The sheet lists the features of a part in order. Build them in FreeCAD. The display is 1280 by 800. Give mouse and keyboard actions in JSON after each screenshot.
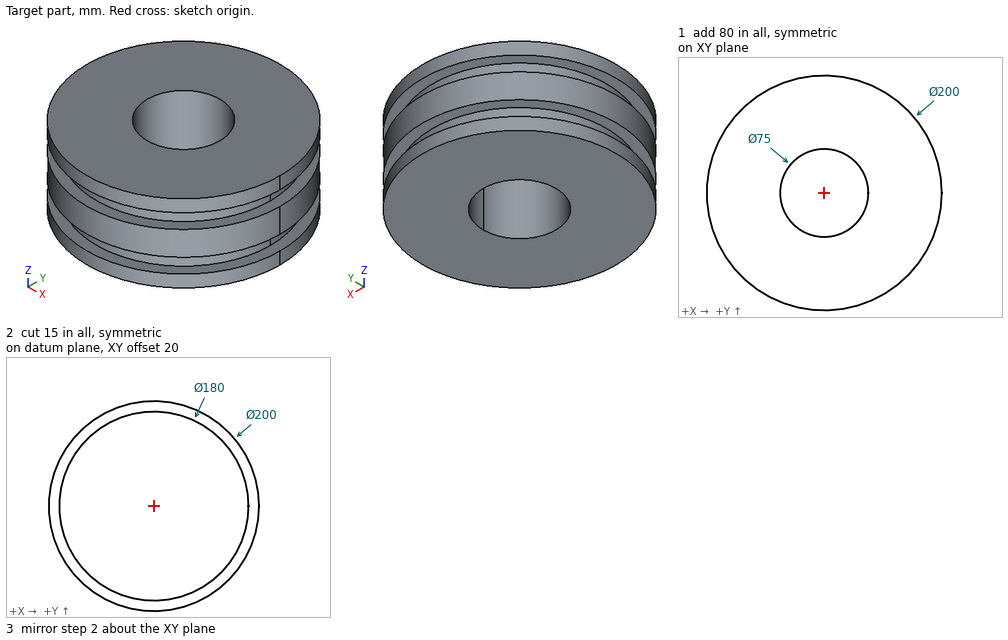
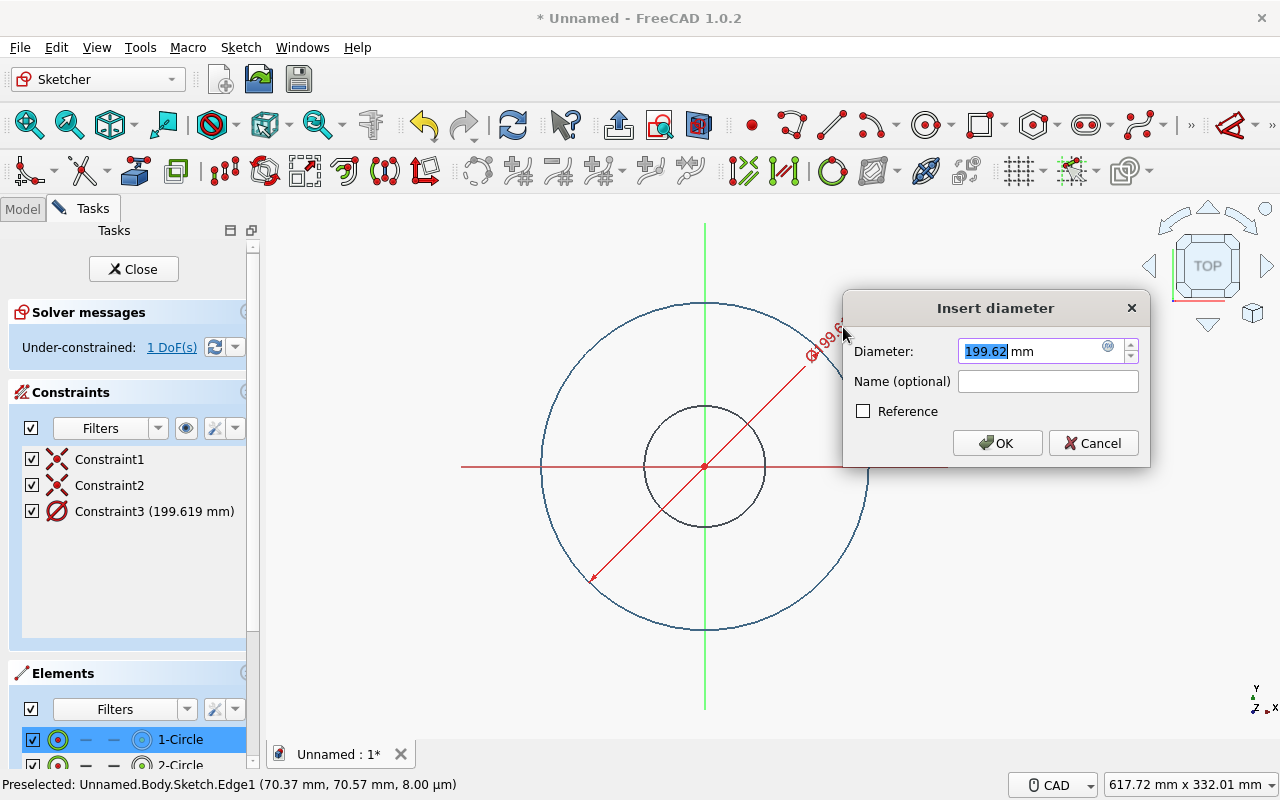
{"action": "type", "text": "200"}
{"action": "key", "text": "Return"}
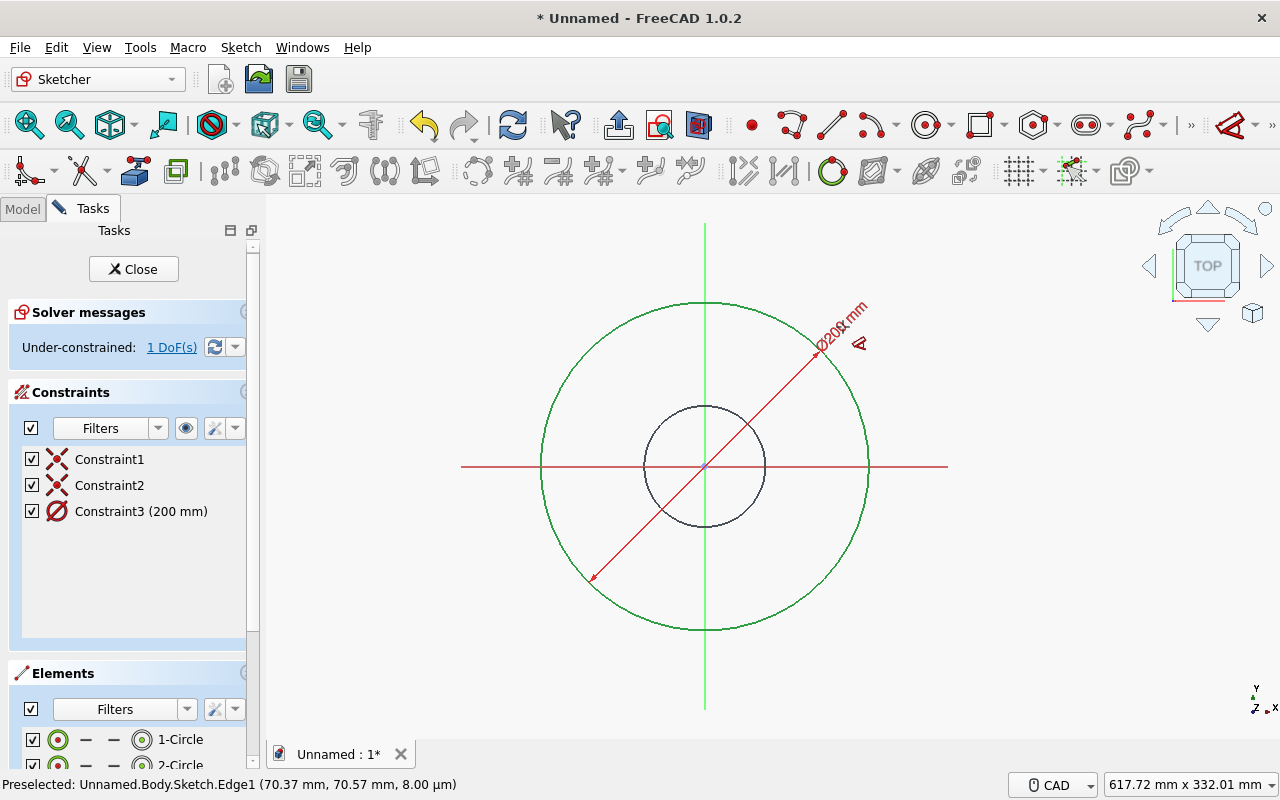
{"action": "left_click", "coordinate": [748, 424]}
{"action": "left_click", "coordinate": [771, 402]}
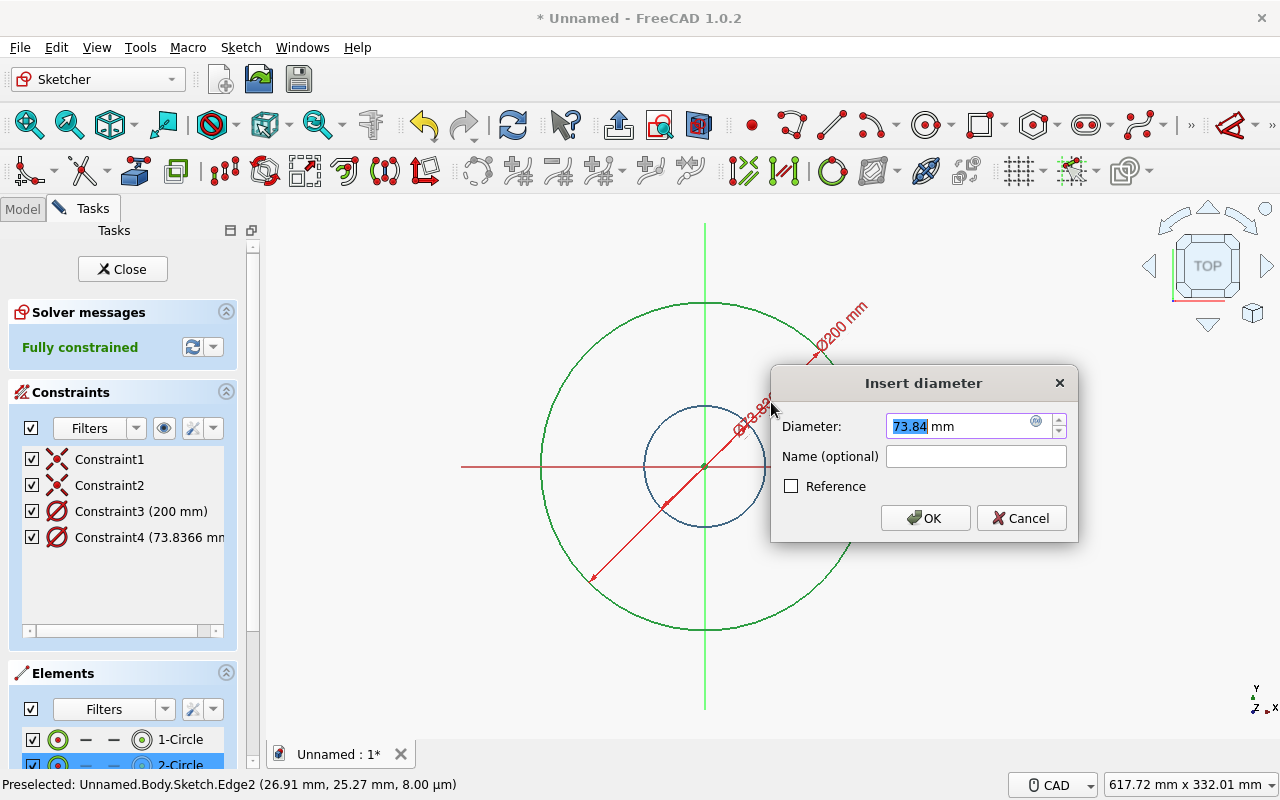
{"action": "type", "text": "75"}
{"action": "key", "text": "Return"}
{"action": "key", "text": "Escape"}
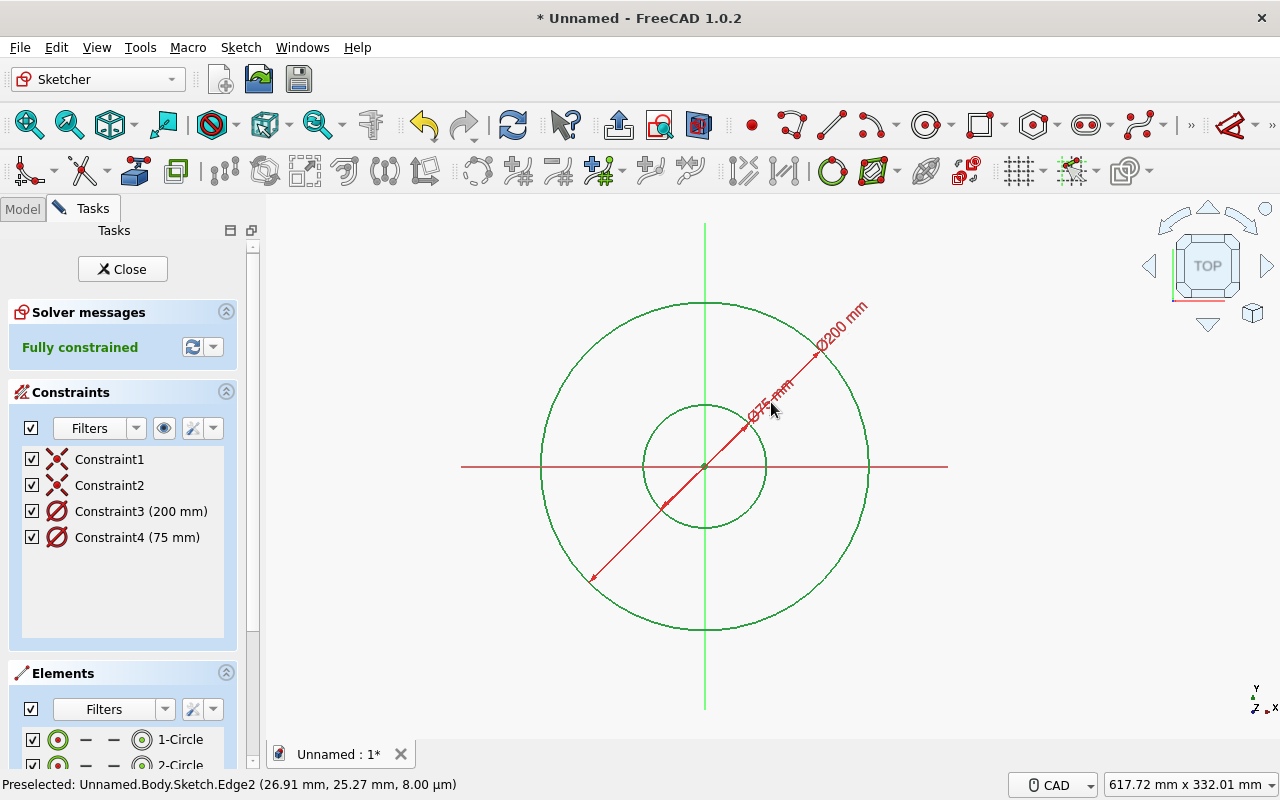
{"action": "left_click", "coordinate": [123, 269]}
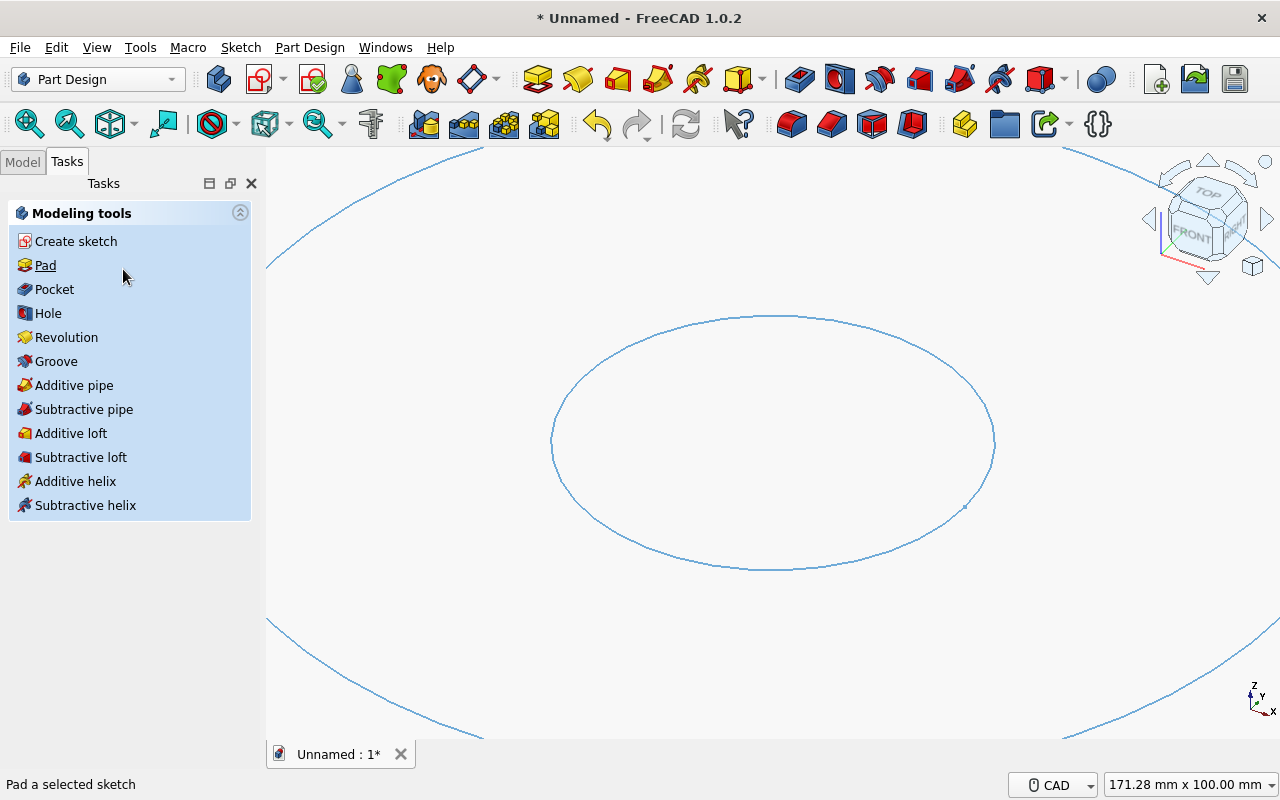
{"action": "left_click", "coordinate": [538, 80]}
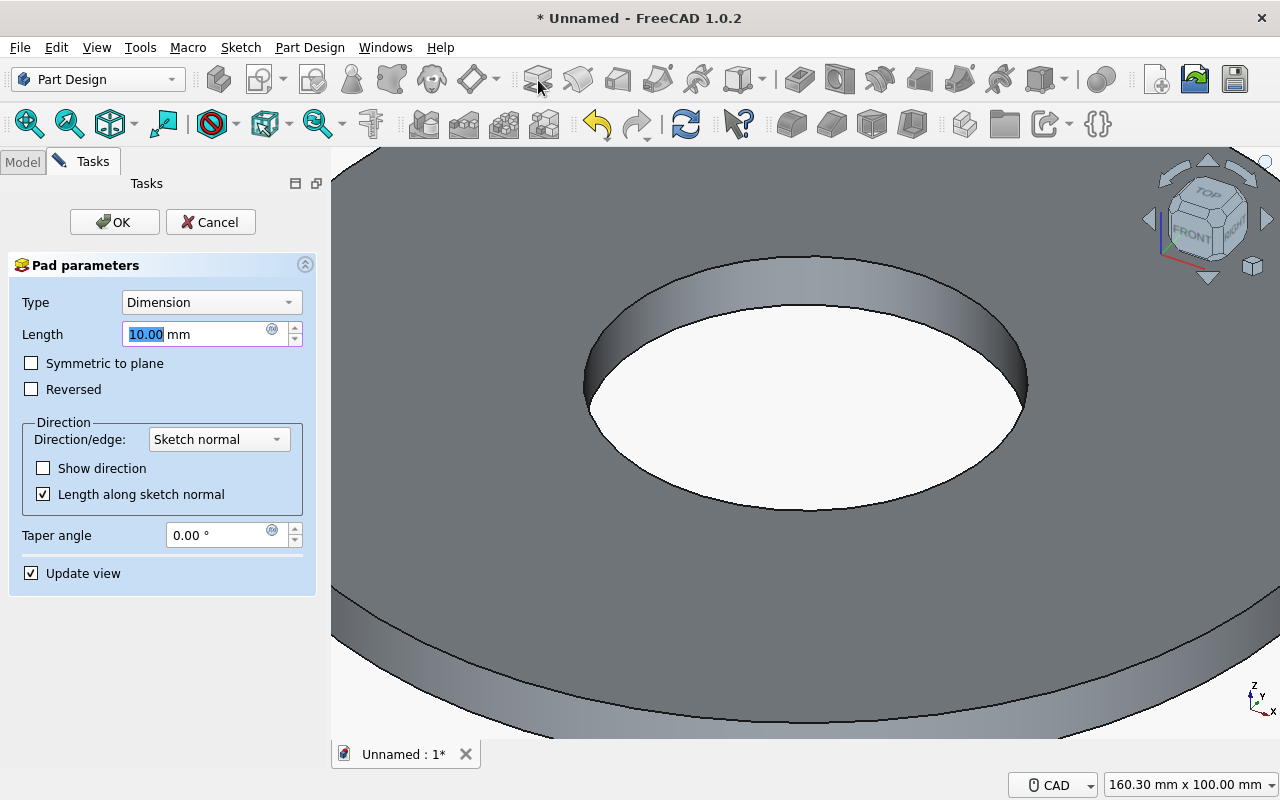
{"action": "type", "text": "80"}
{"action": "key", "text": "Tab"}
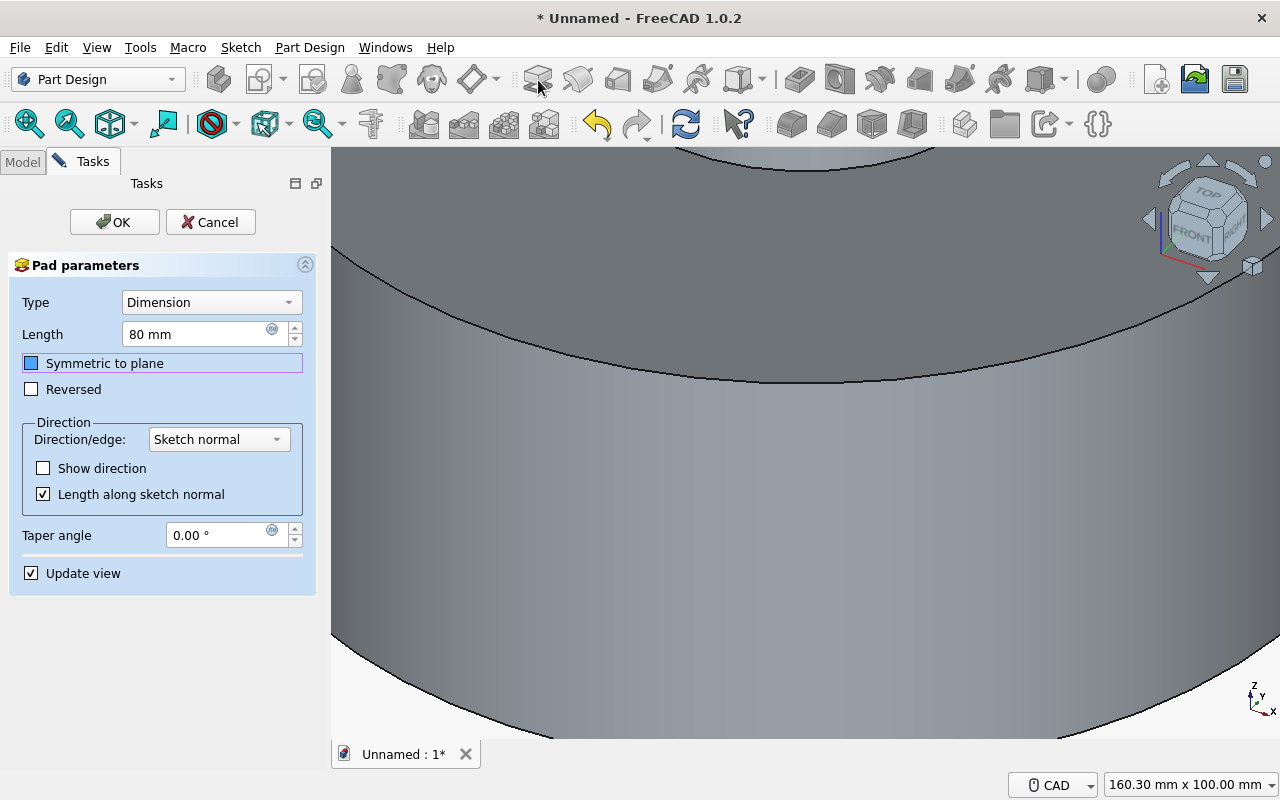
{"action": "left_click", "coordinate": [30, 363]}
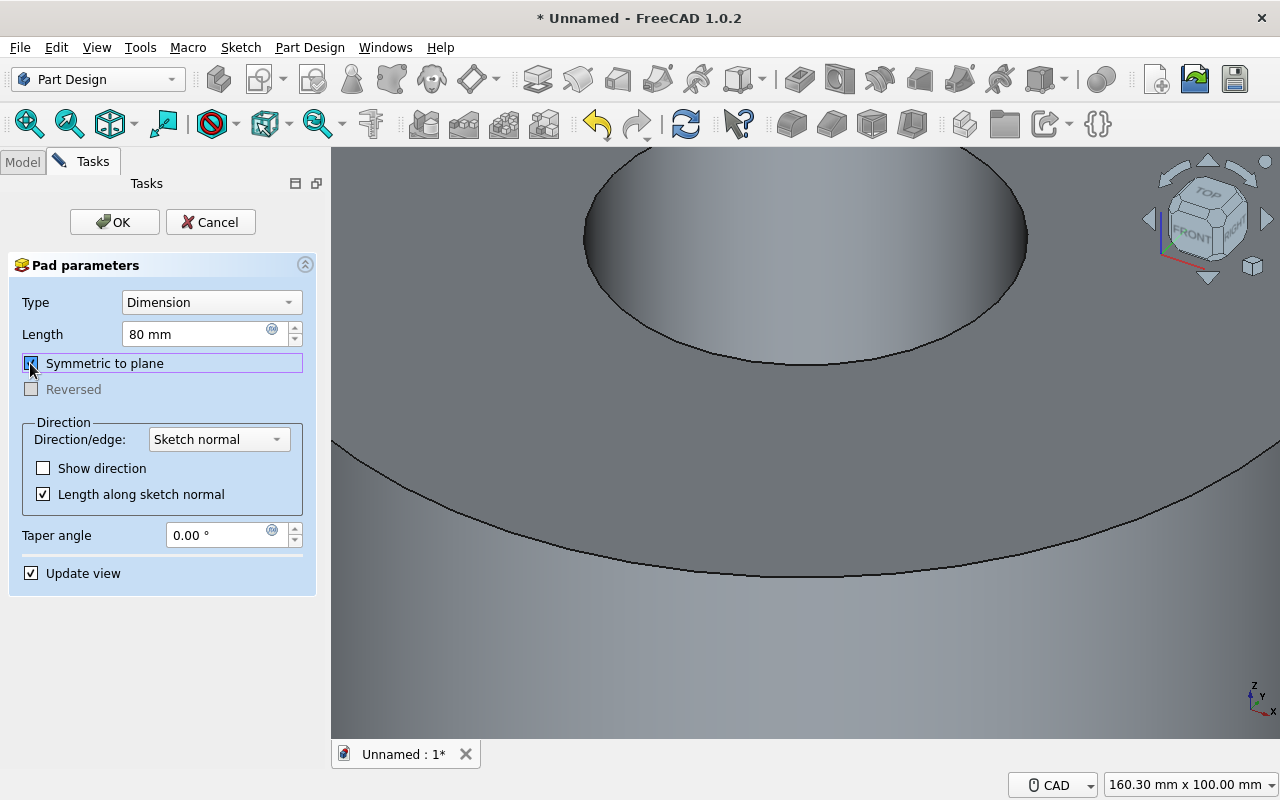
{"action": "left_click", "coordinate": [115, 222]}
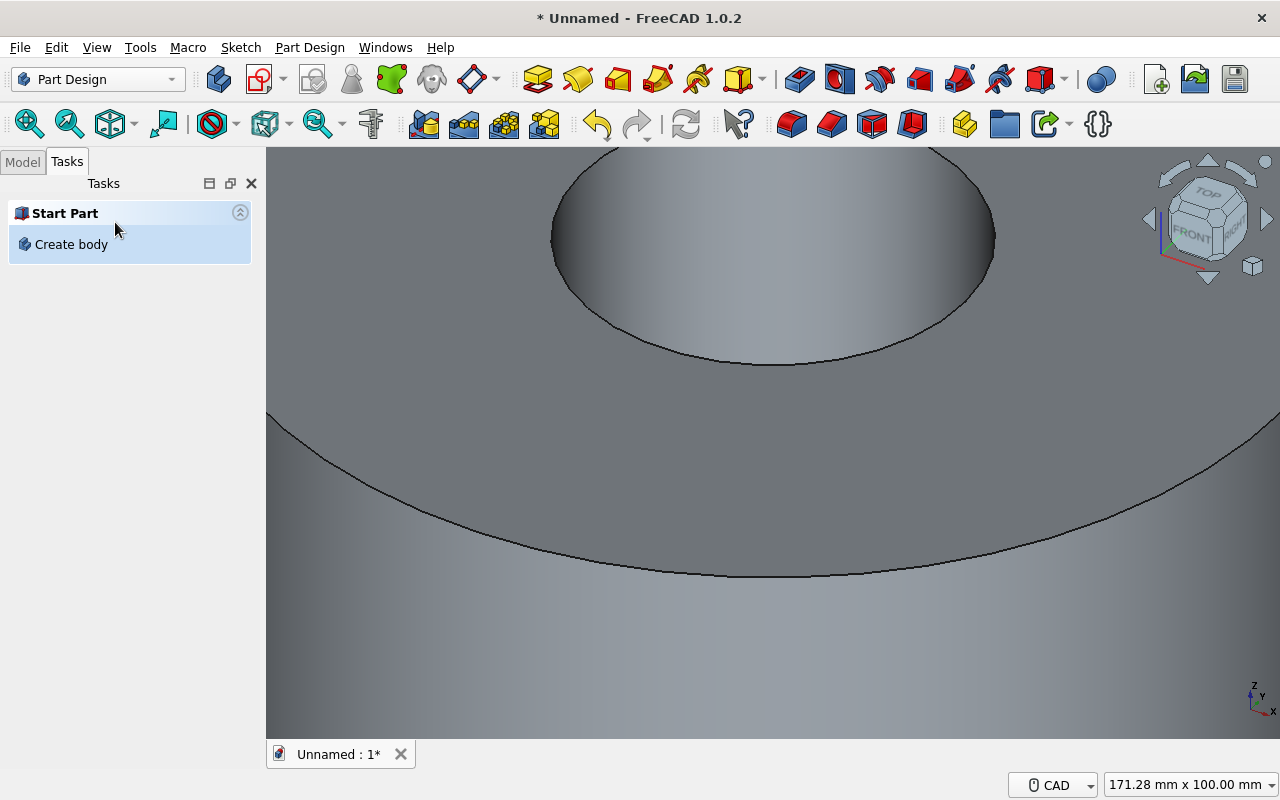
{"action": "left_click", "coordinate": [30, 124]}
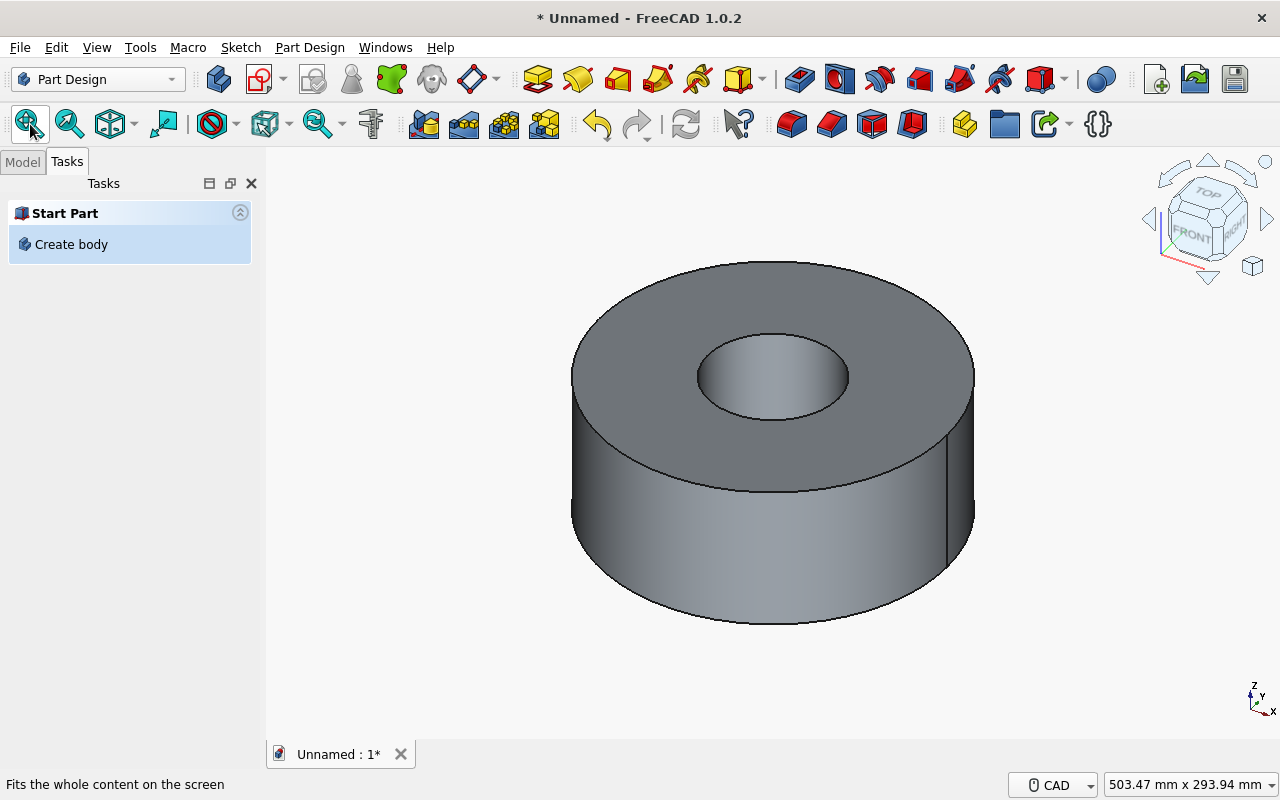
{"action": "left_click", "coordinate": [23, 161]}